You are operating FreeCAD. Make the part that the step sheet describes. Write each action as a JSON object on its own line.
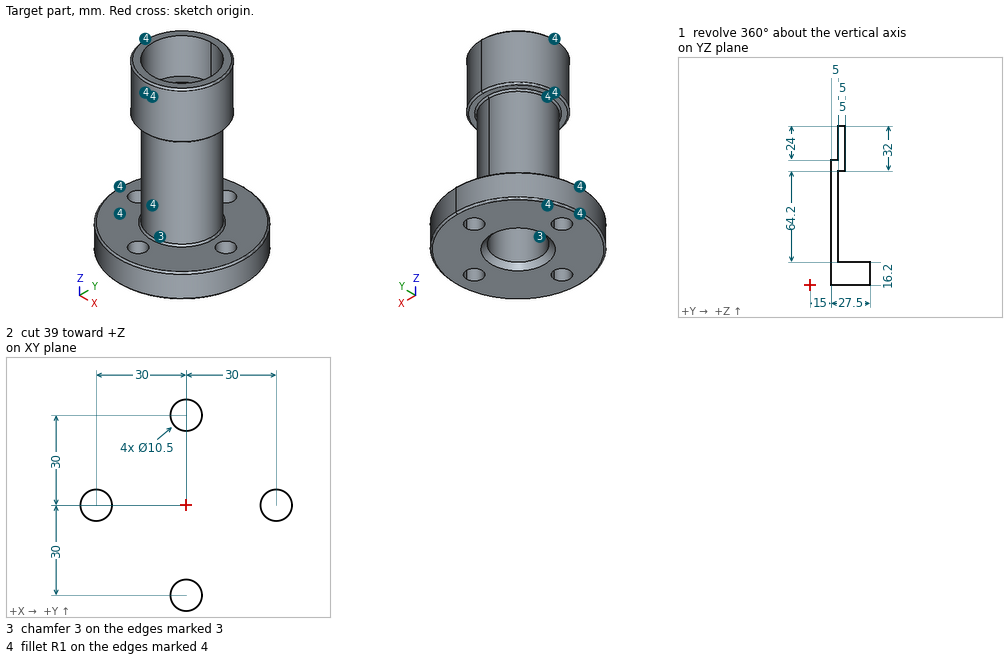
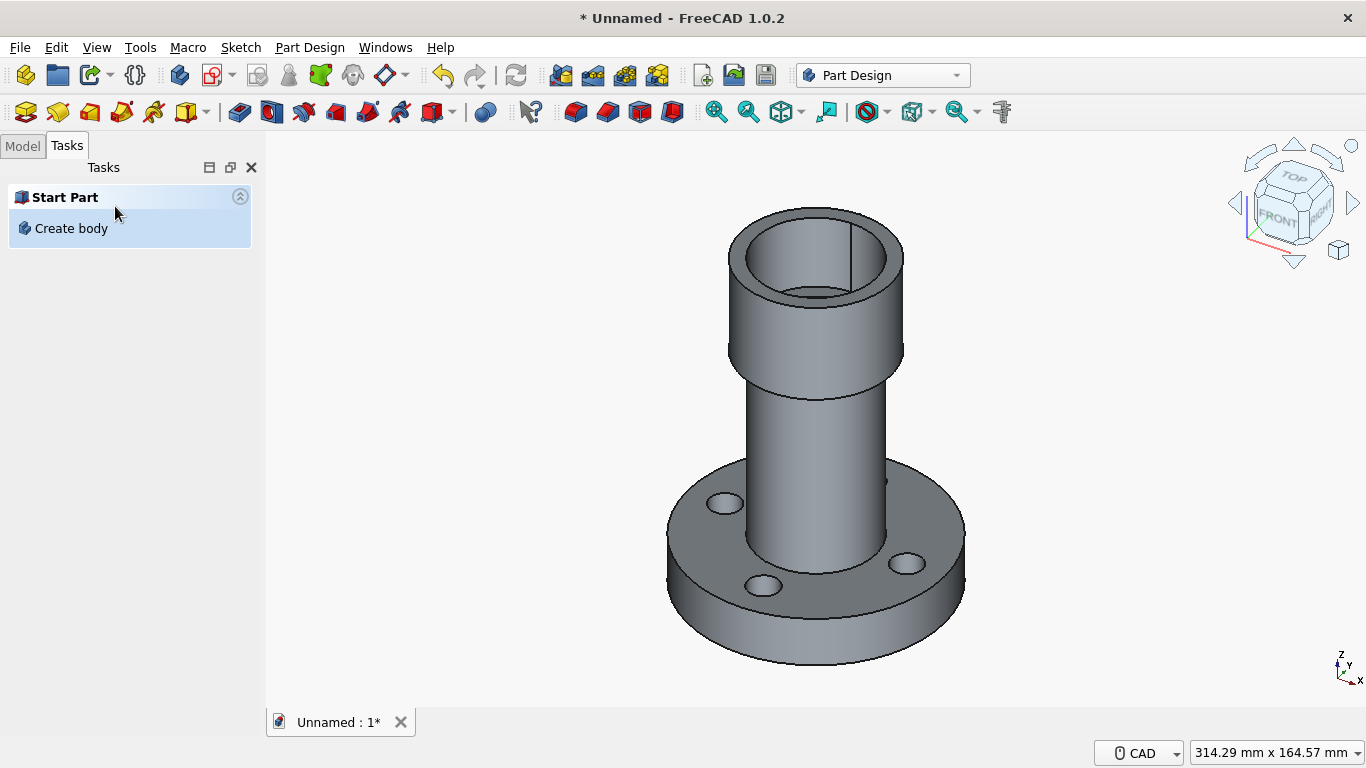
{"action": "key", "text": "0"}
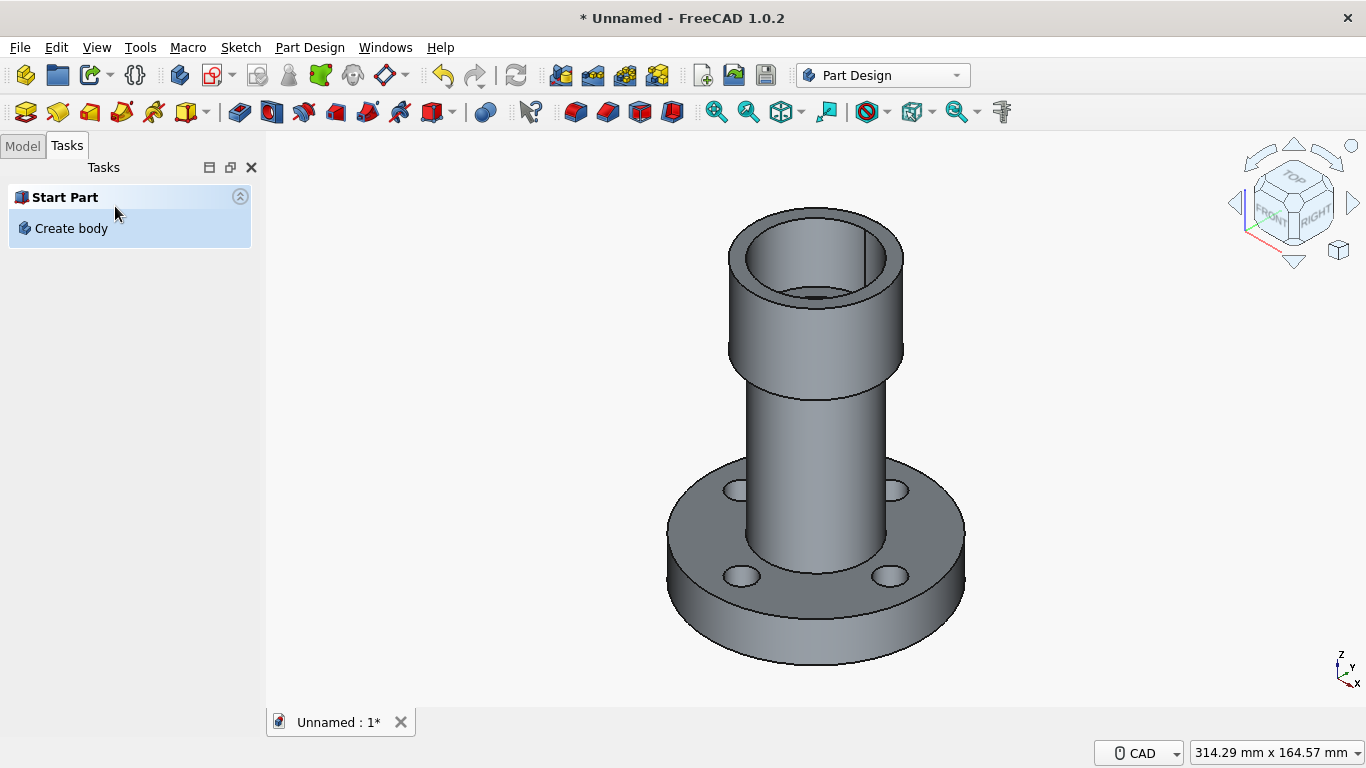
{"action": "key", "text": "2"}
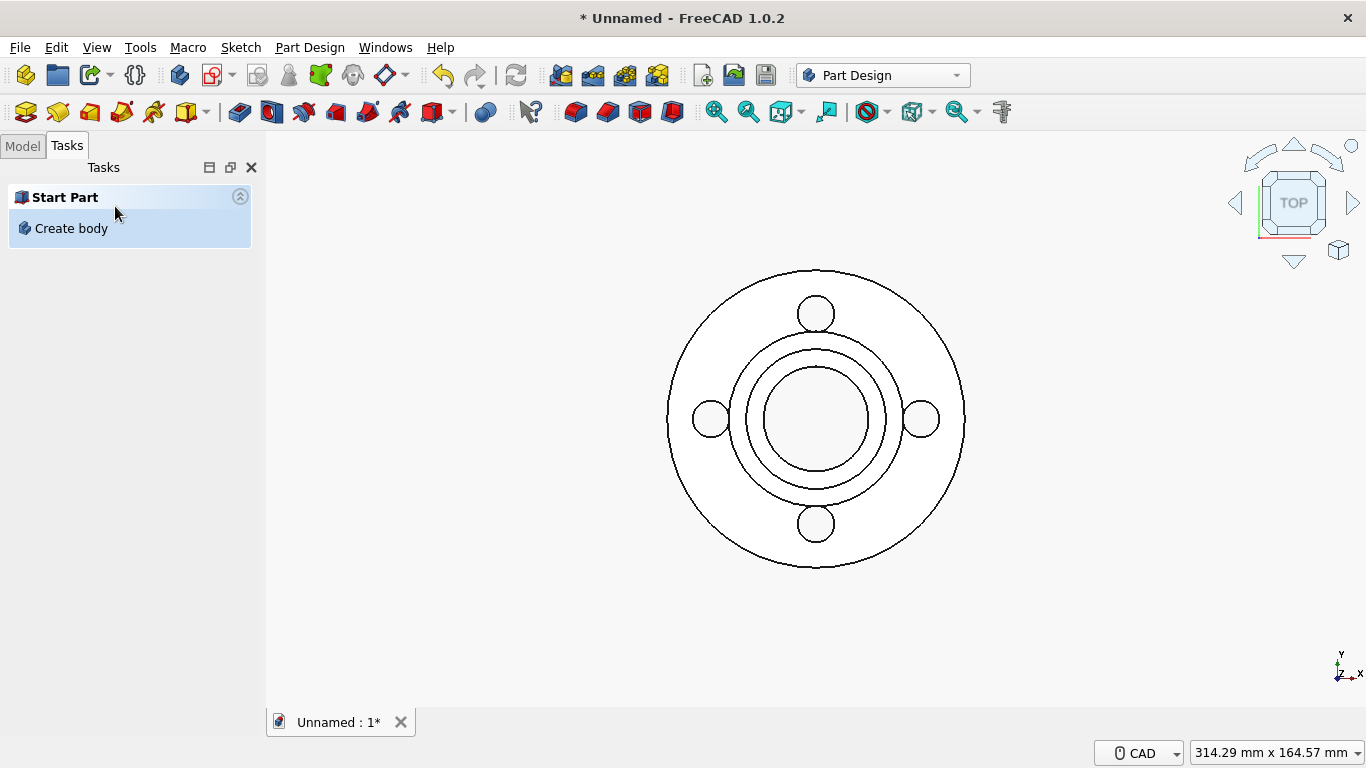
{"action": "key", "text": "1"}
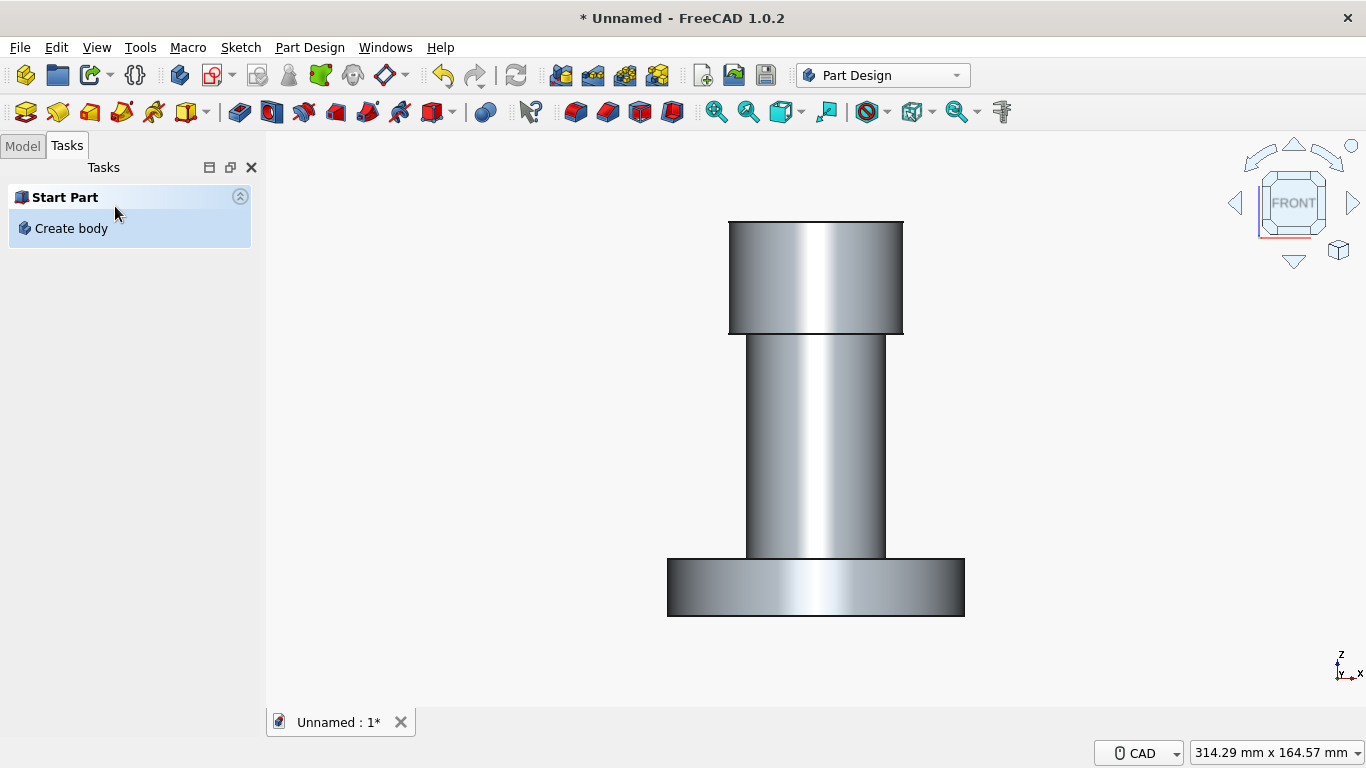
{"action": "key", "text": "3"}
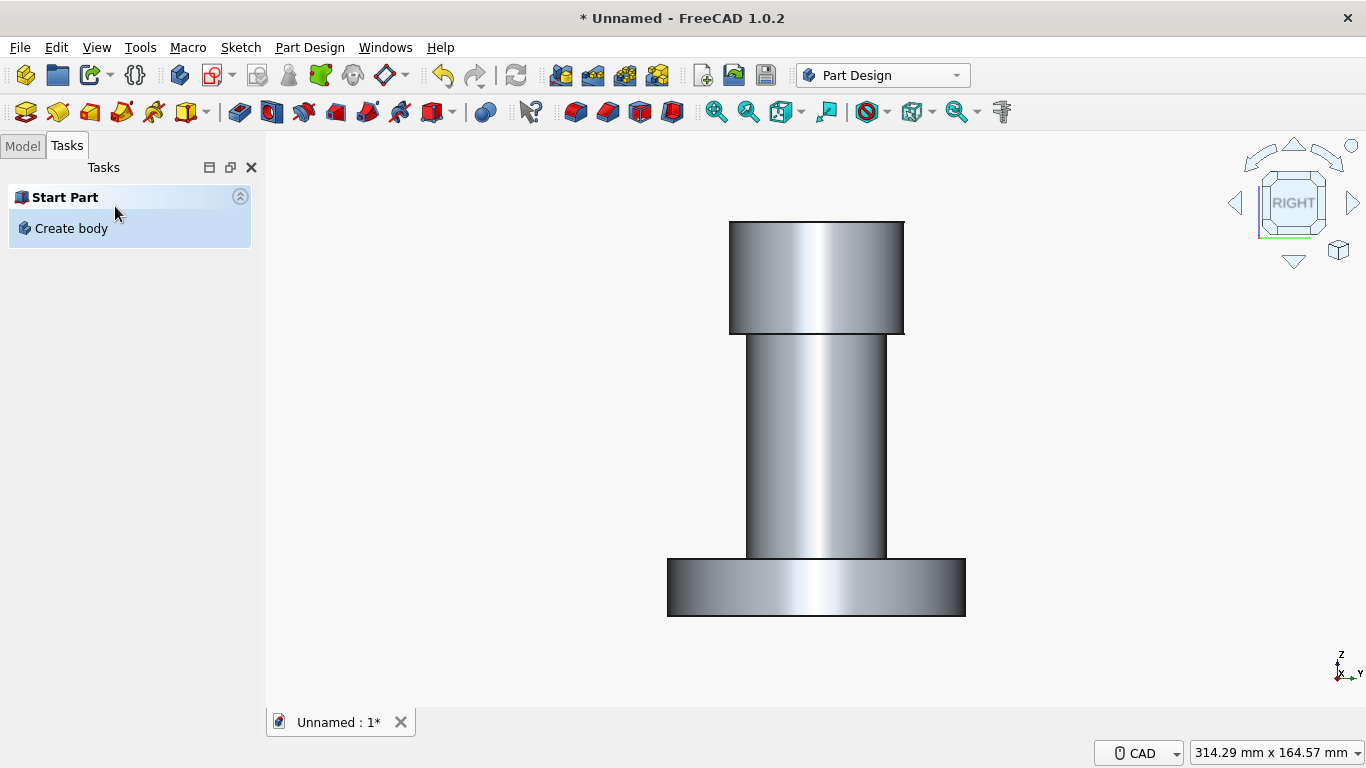
{"action": "key", "text": "5"}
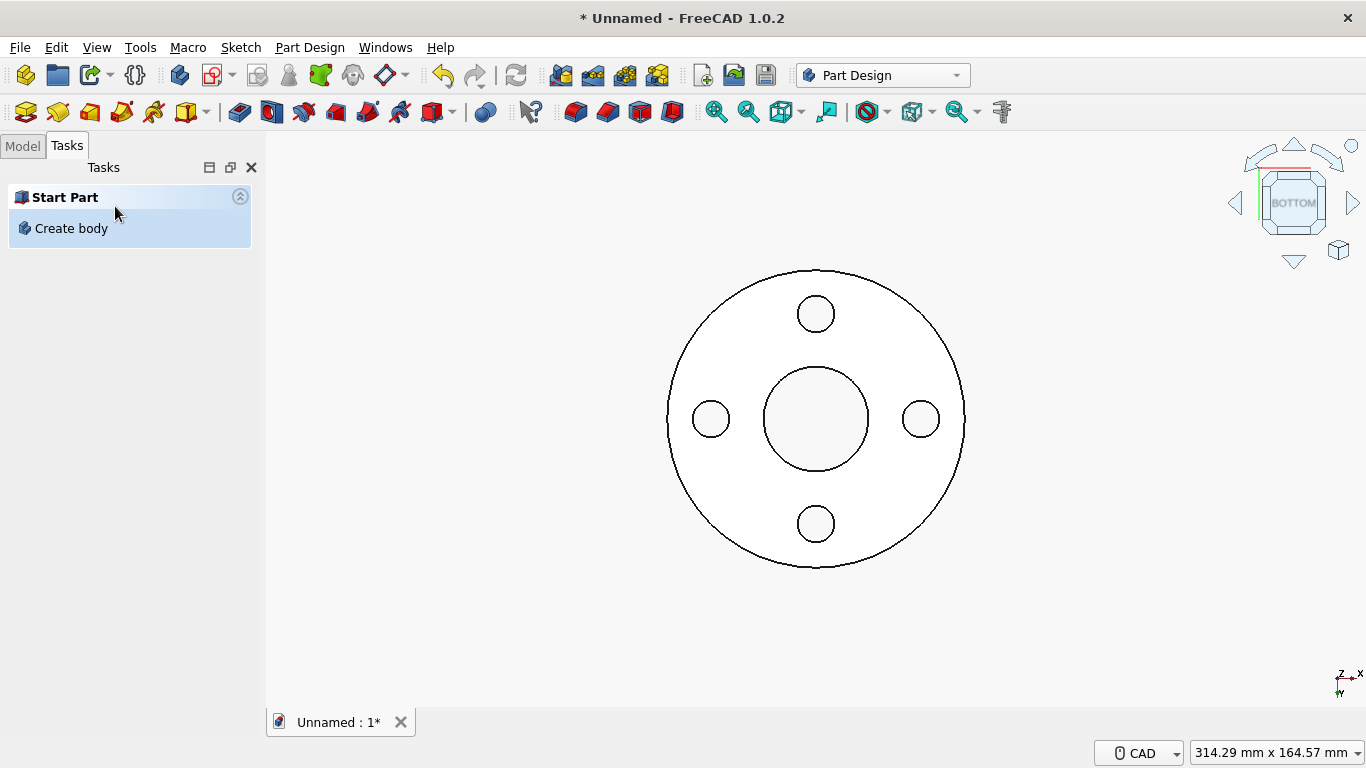
{"action": "left_click", "coordinate": [816, 366]}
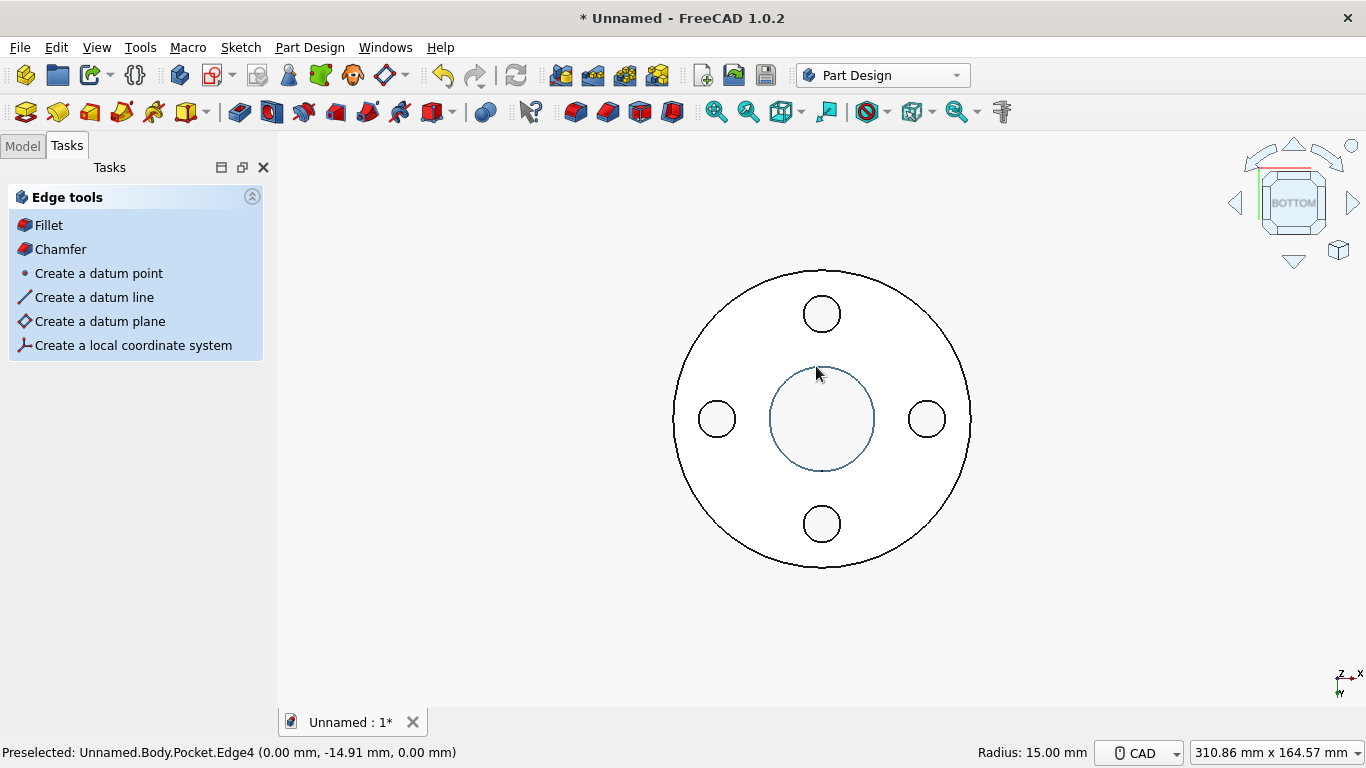
{"action": "left_click", "coordinate": [608, 112]}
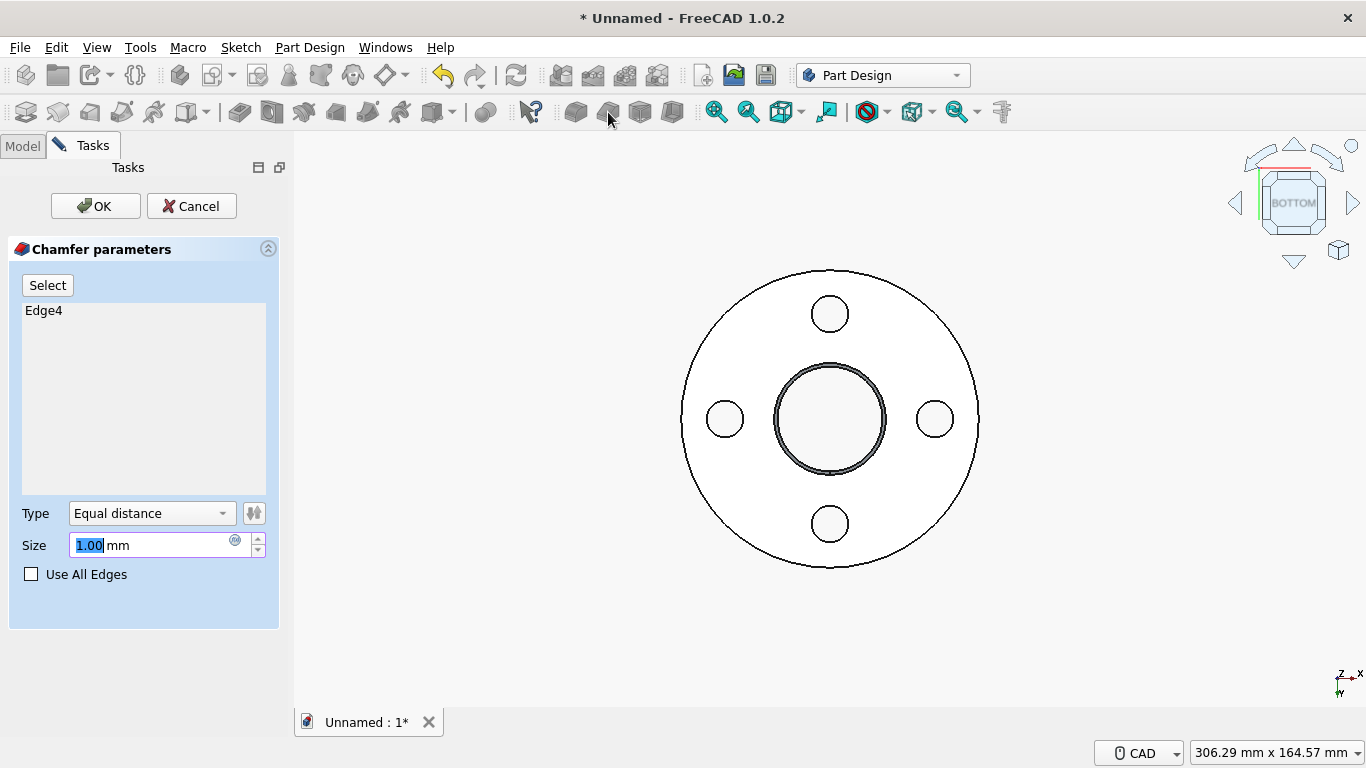
{"action": "type", "text": "3"}
{"action": "key", "text": "Tab"}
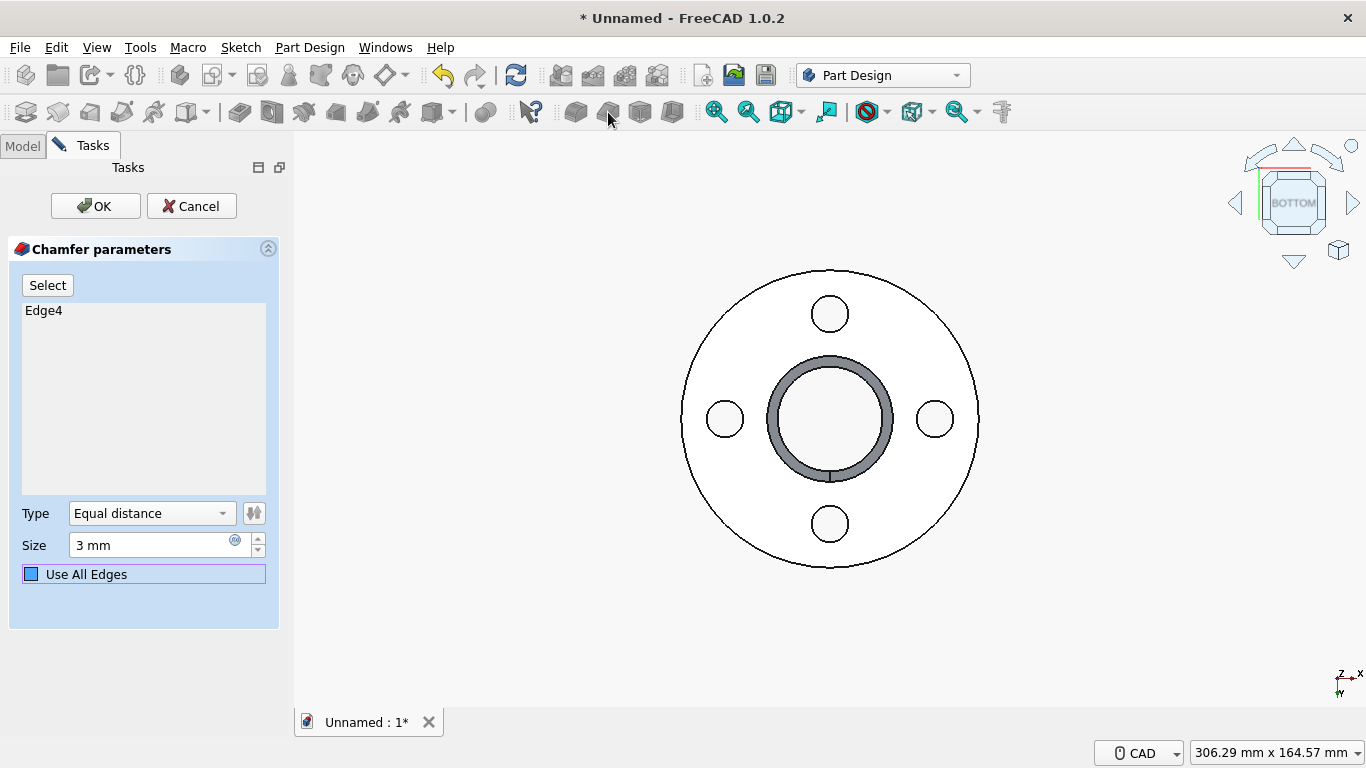
{"action": "left_click", "coordinate": [96, 206]}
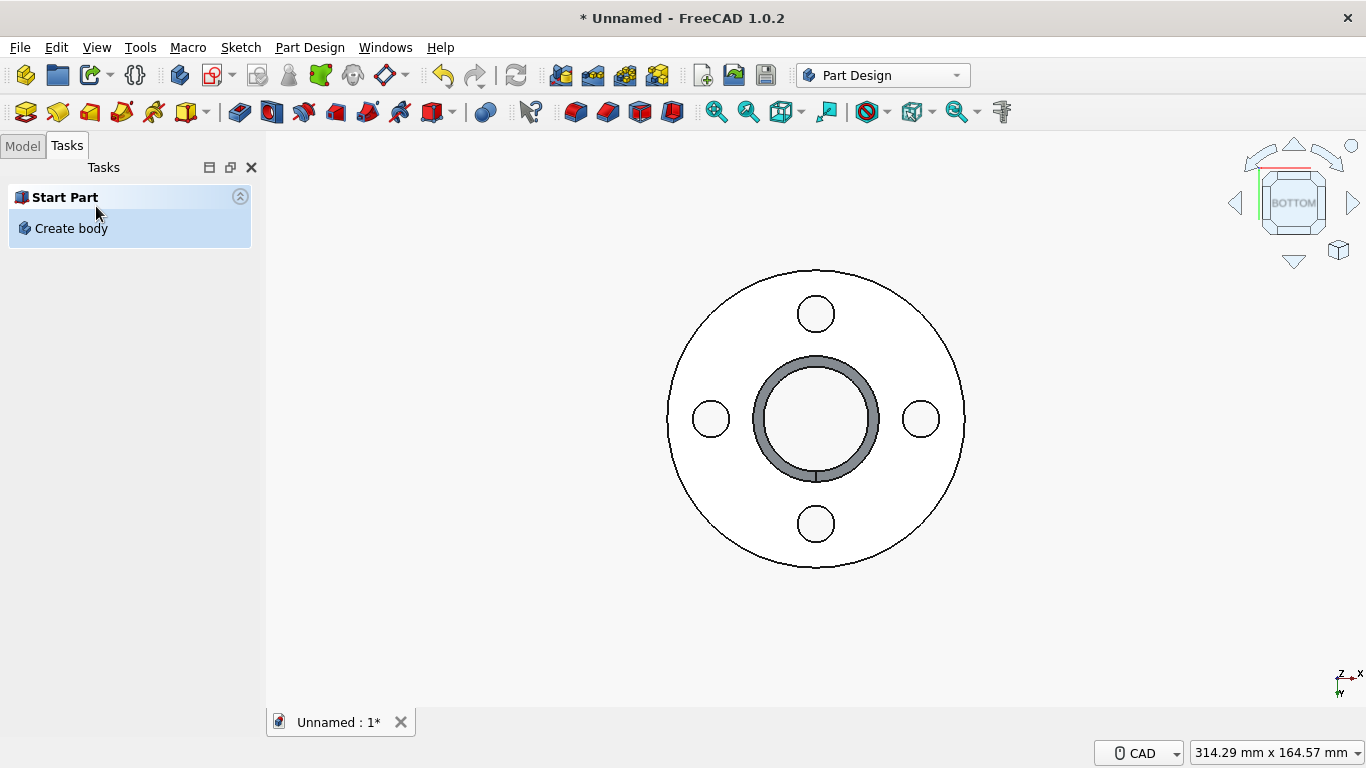
{"action": "left_click", "coordinate": [816, 269]}